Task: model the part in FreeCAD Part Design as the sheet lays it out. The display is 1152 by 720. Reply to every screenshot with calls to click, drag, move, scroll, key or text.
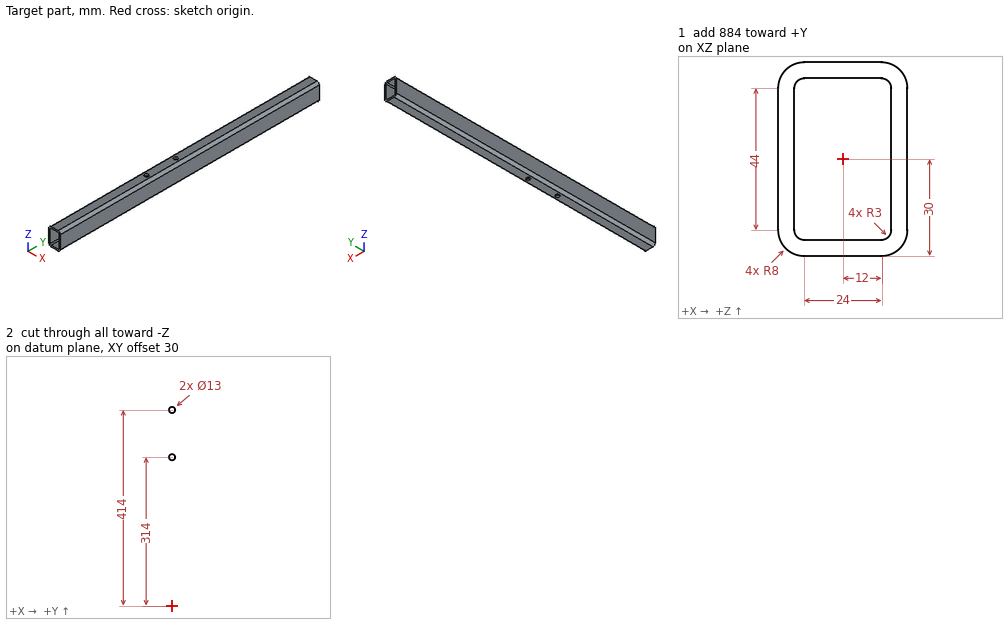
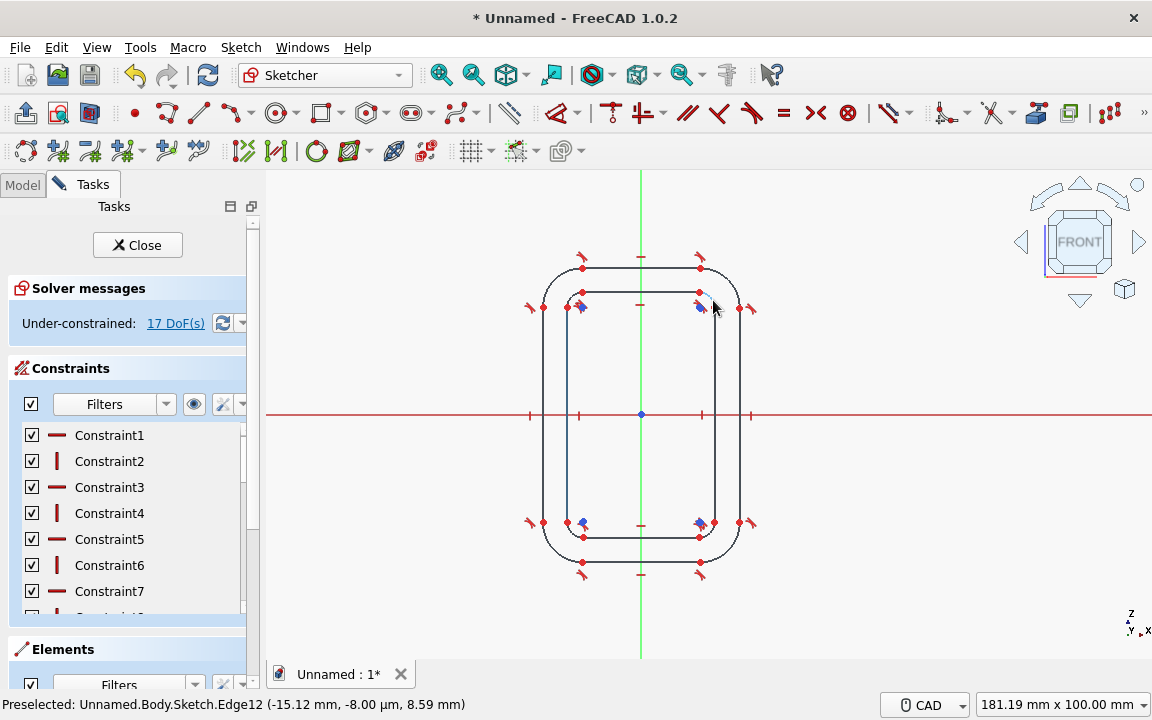
scroll(569, 529, up, 4)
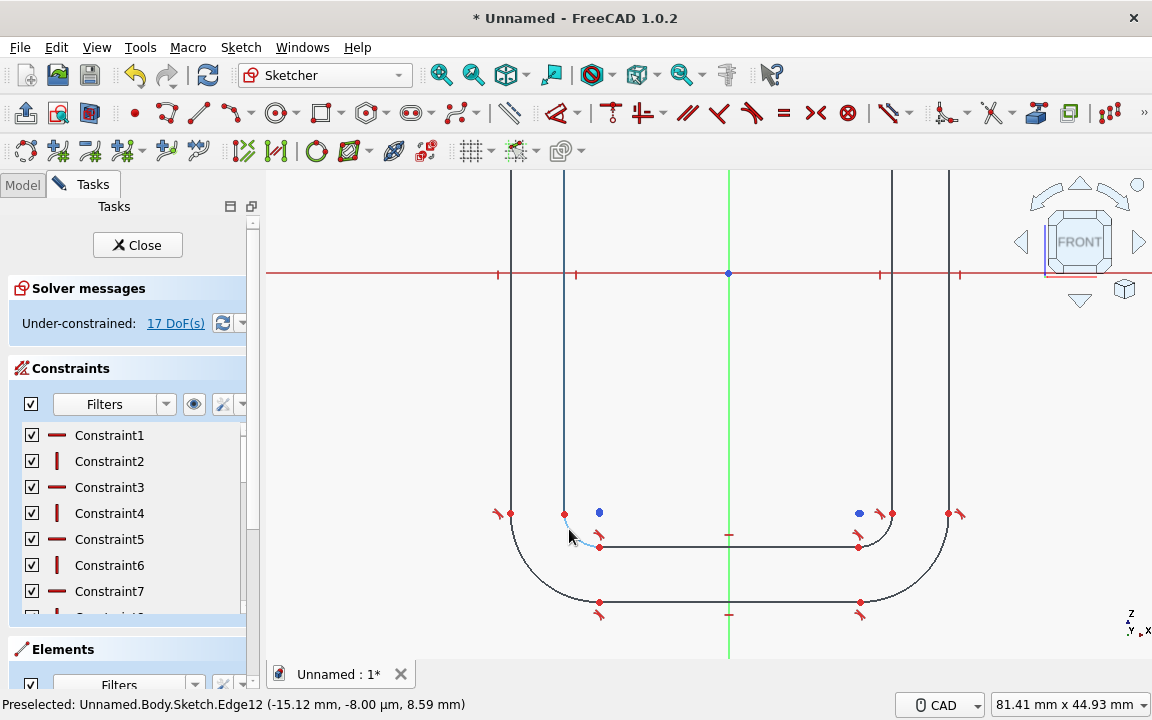
click(569, 529)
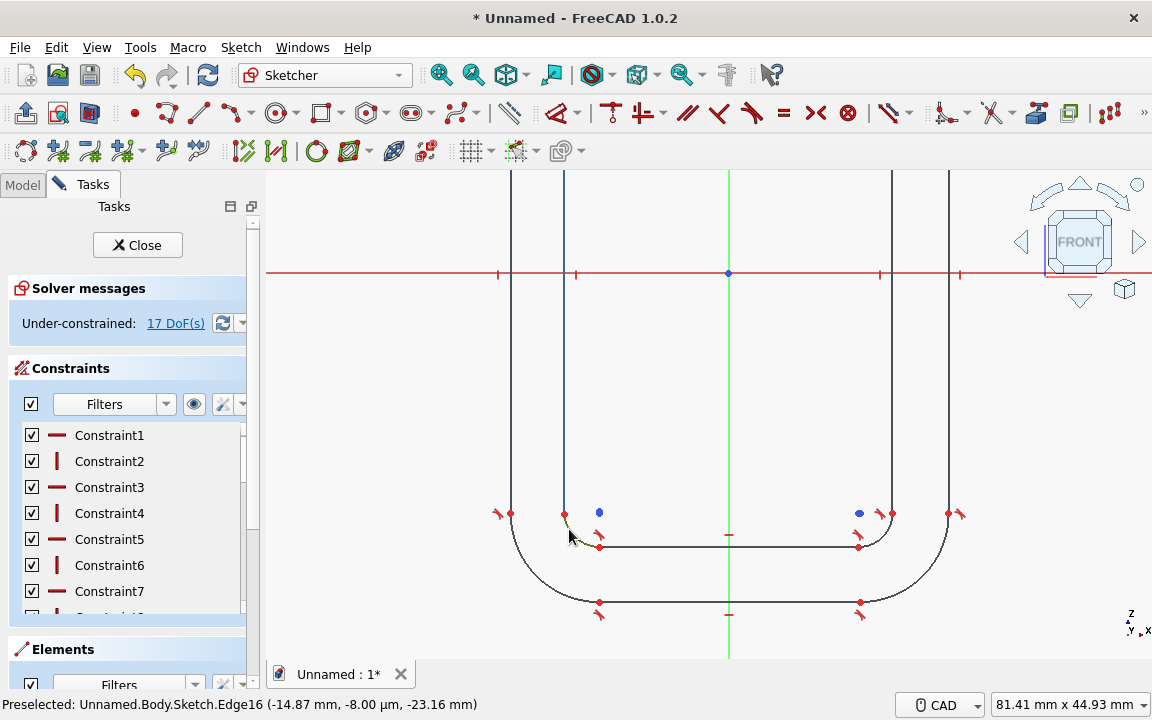
key(t)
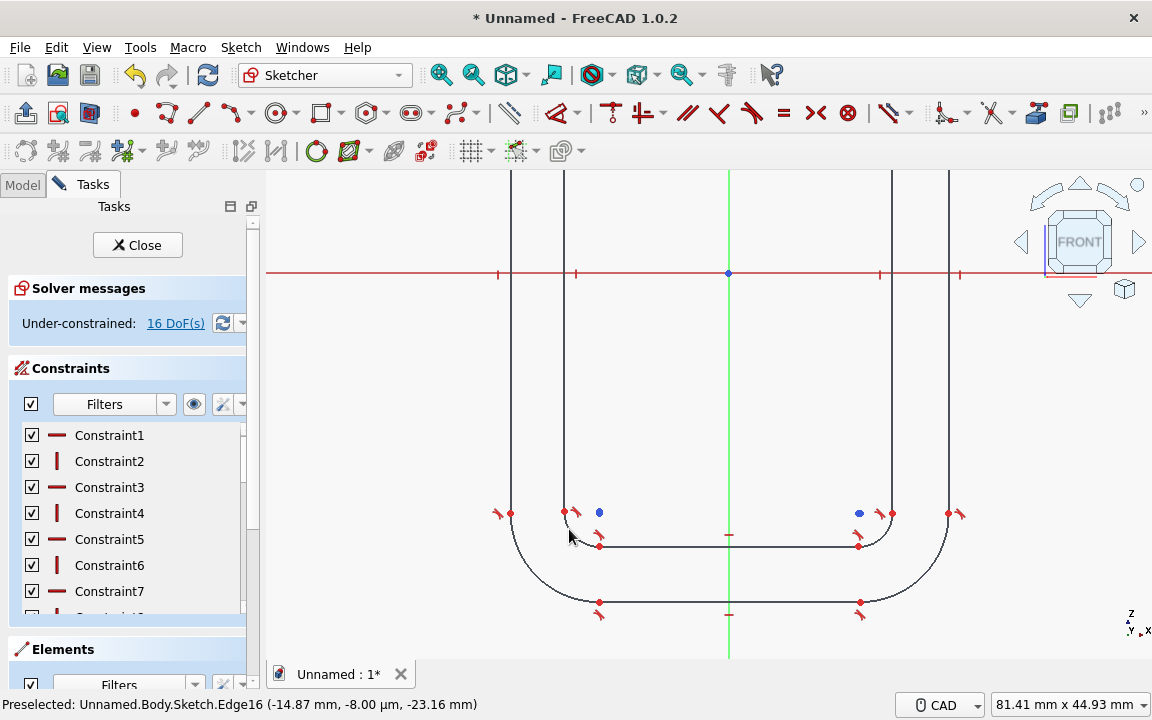
click(900, 592)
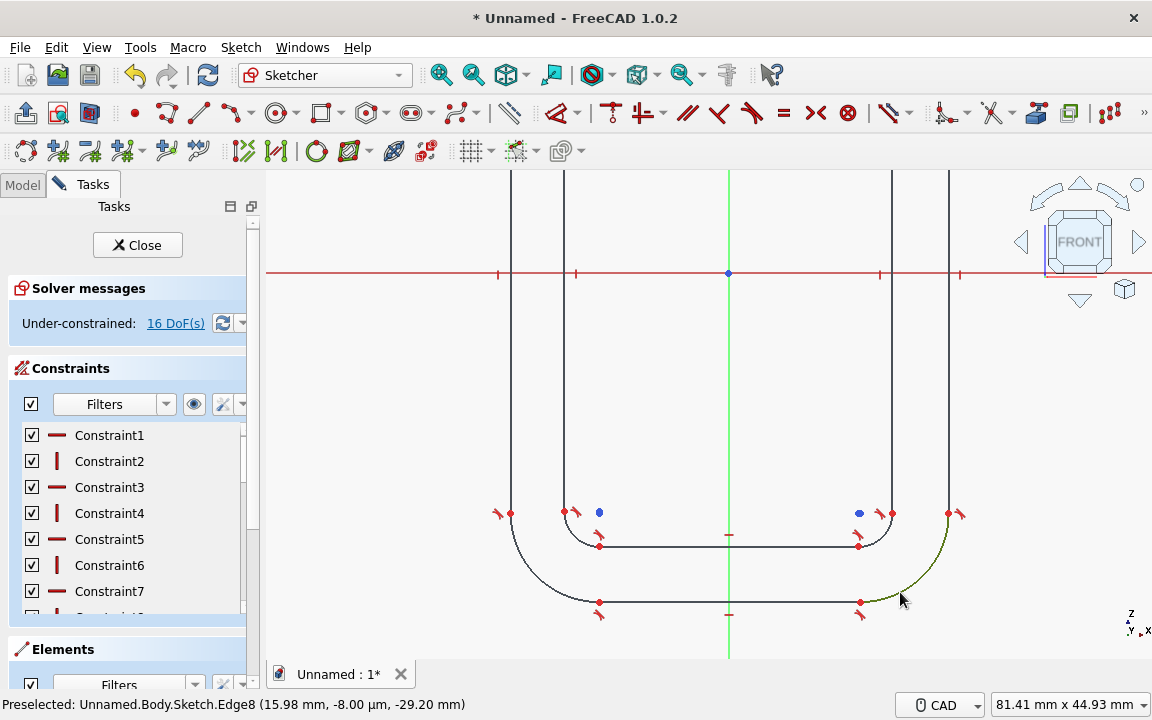
click(874, 543)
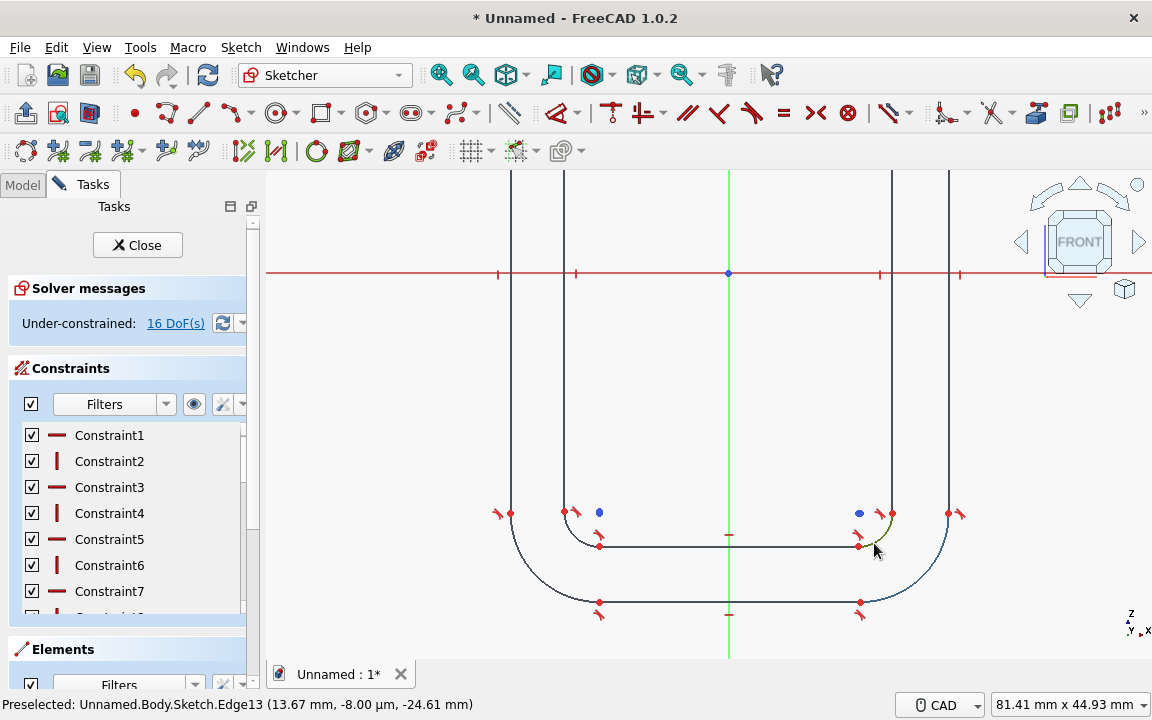
key(c)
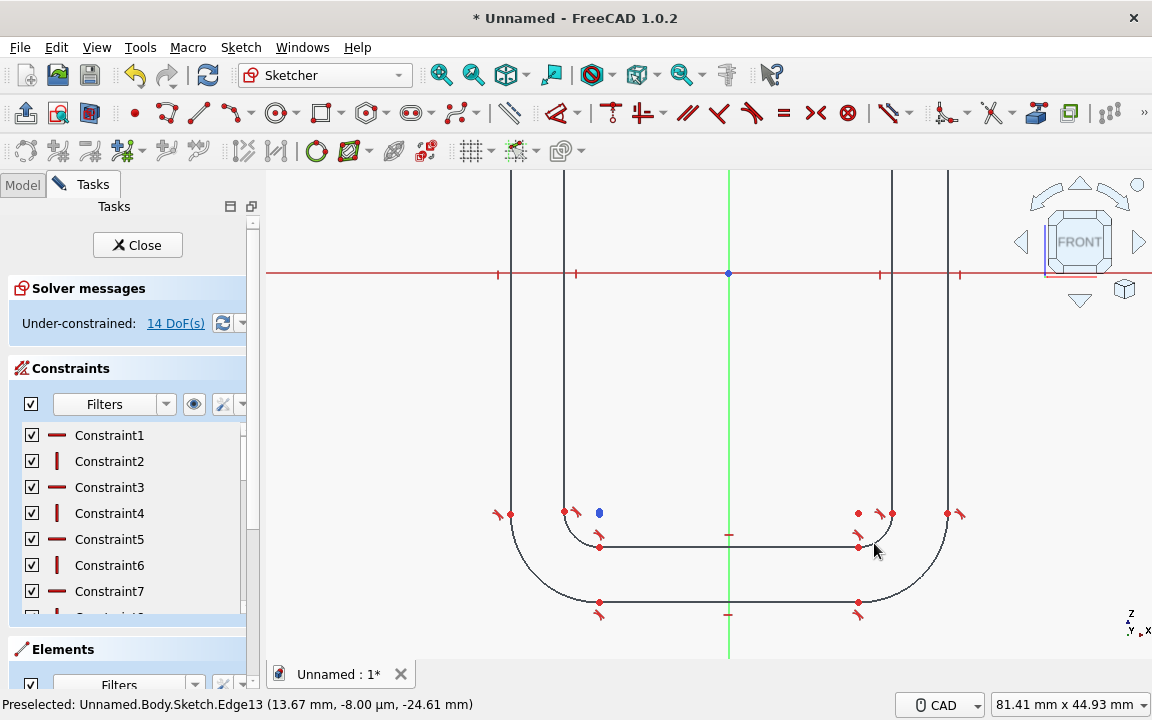
scroll(568, 530, down, 4)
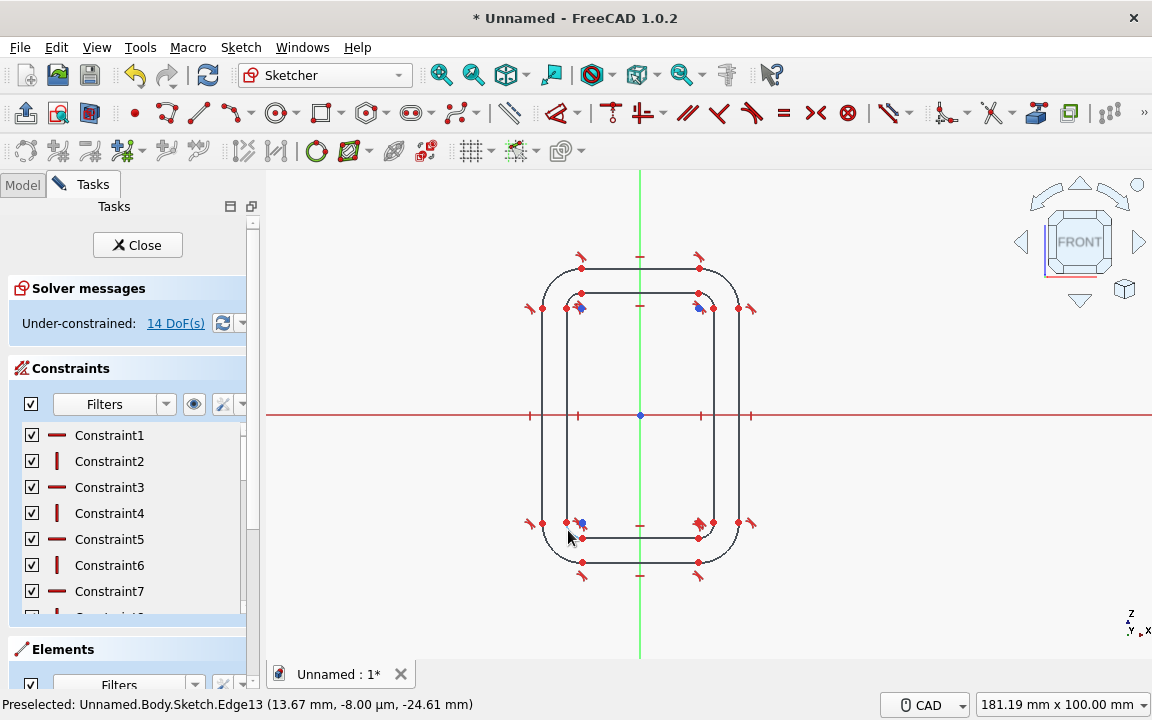
click(735, 291)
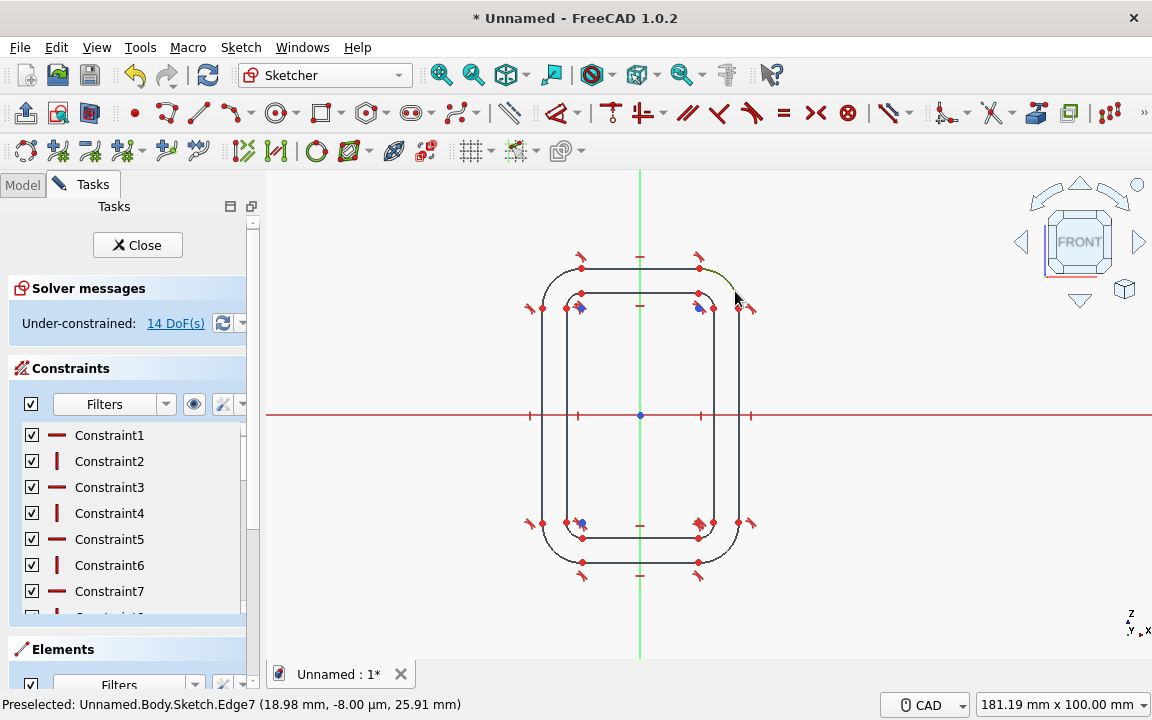
click(710, 297)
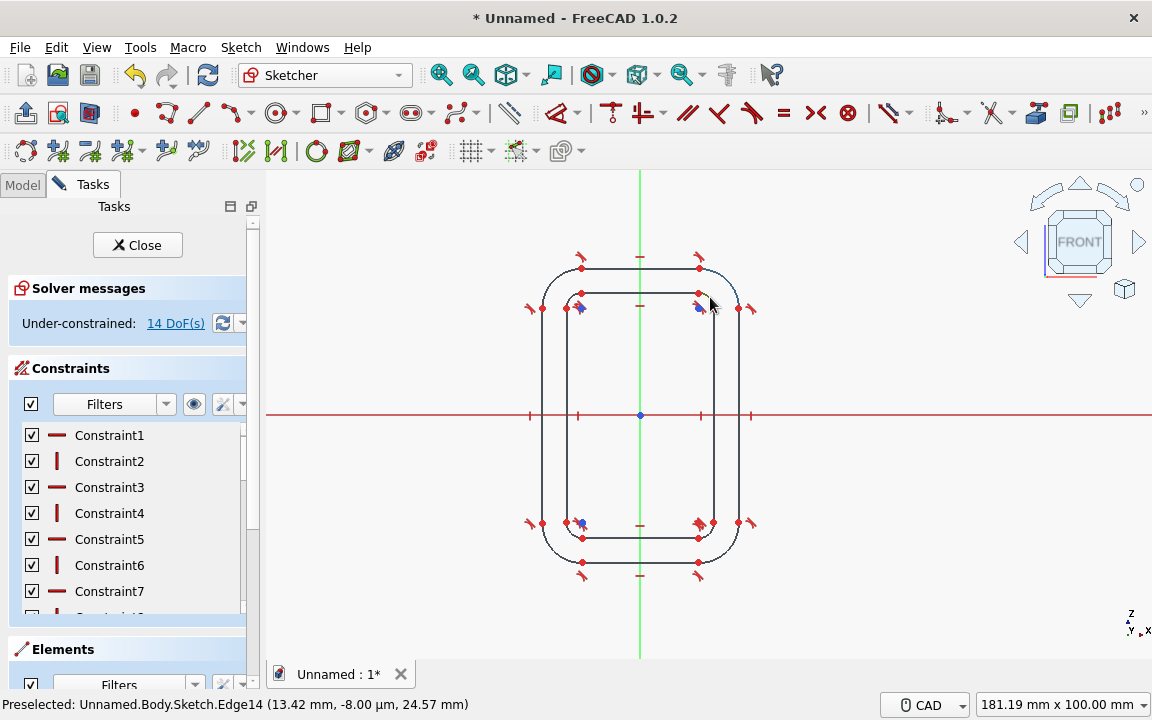
key(c)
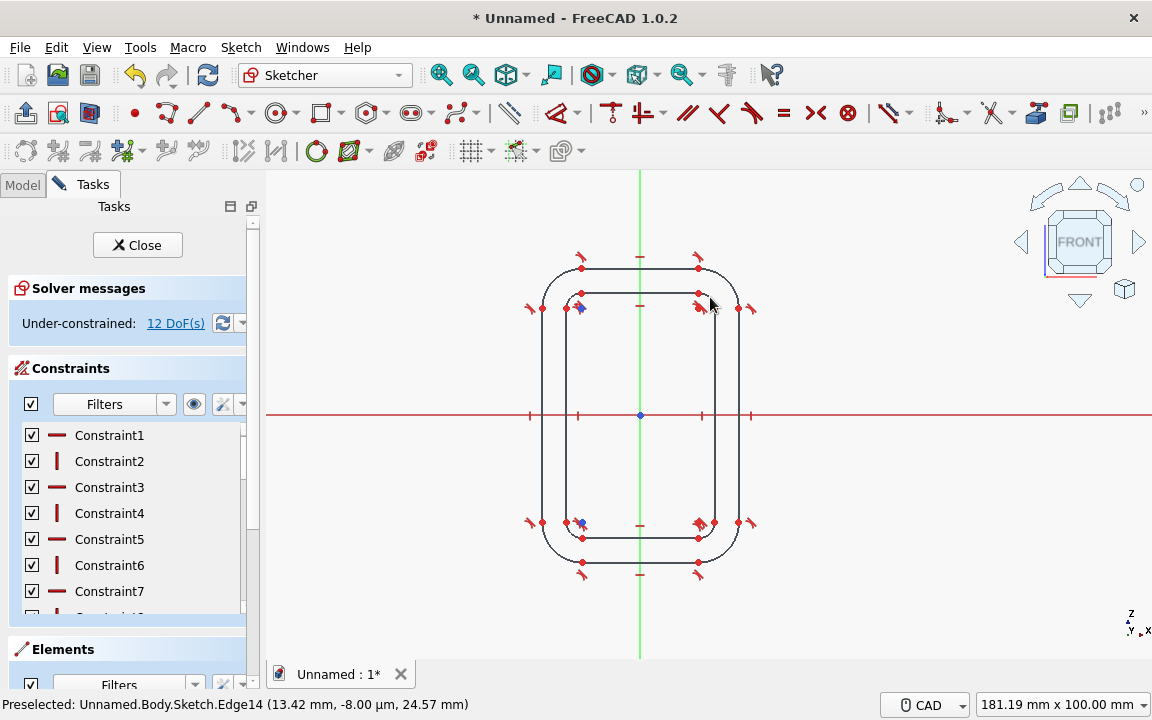
click(564, 273)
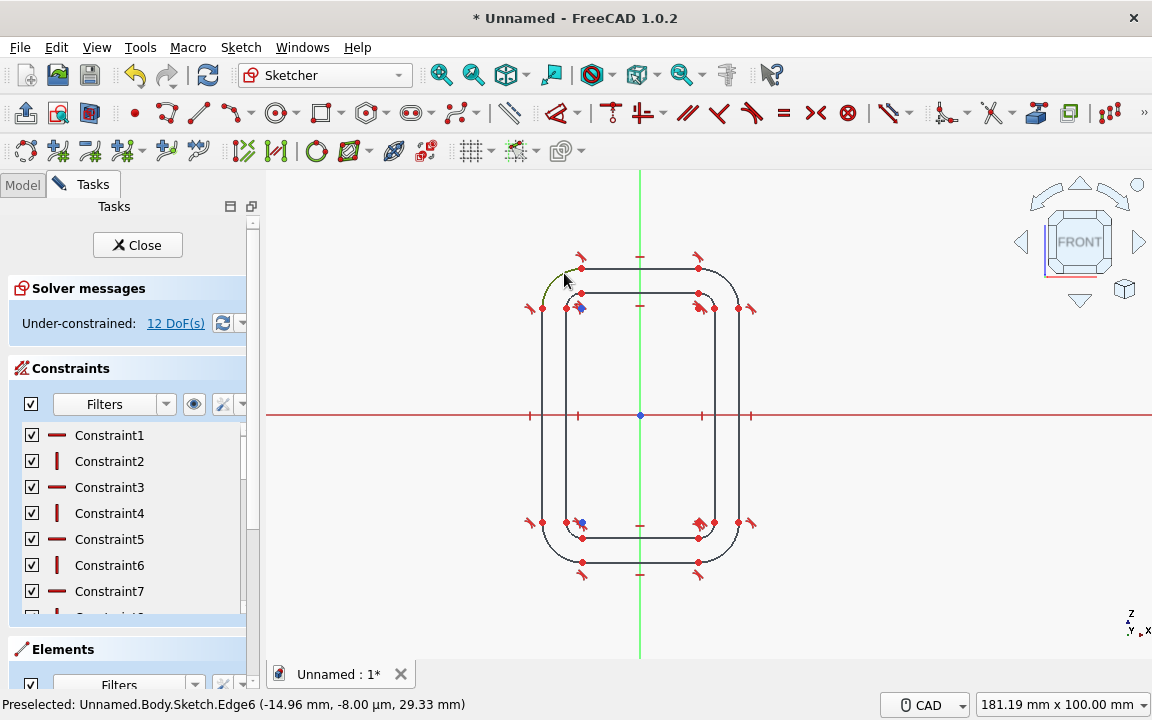
click(571, 298)